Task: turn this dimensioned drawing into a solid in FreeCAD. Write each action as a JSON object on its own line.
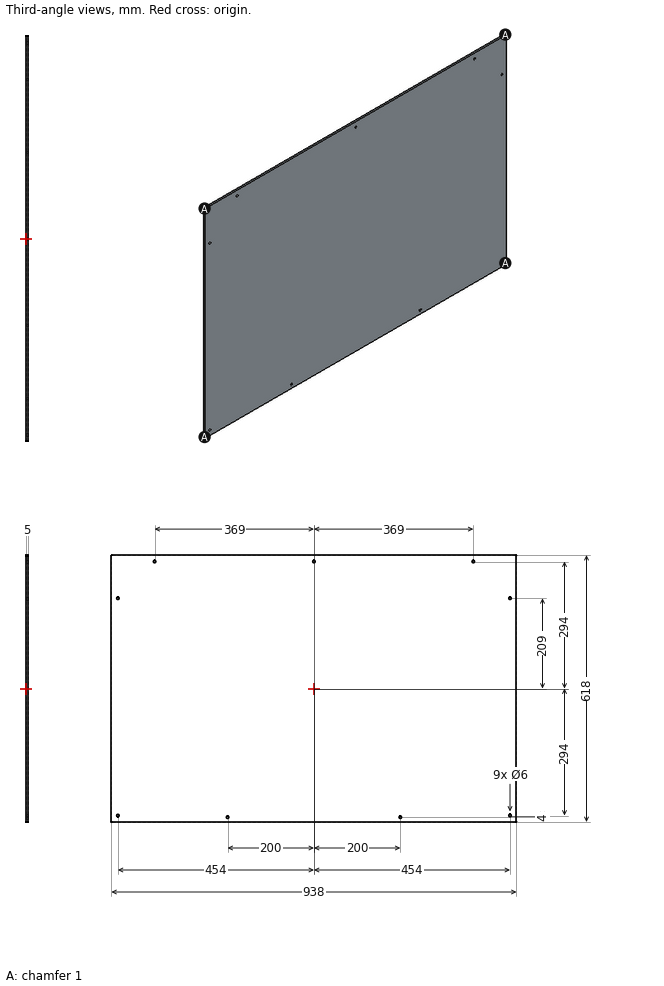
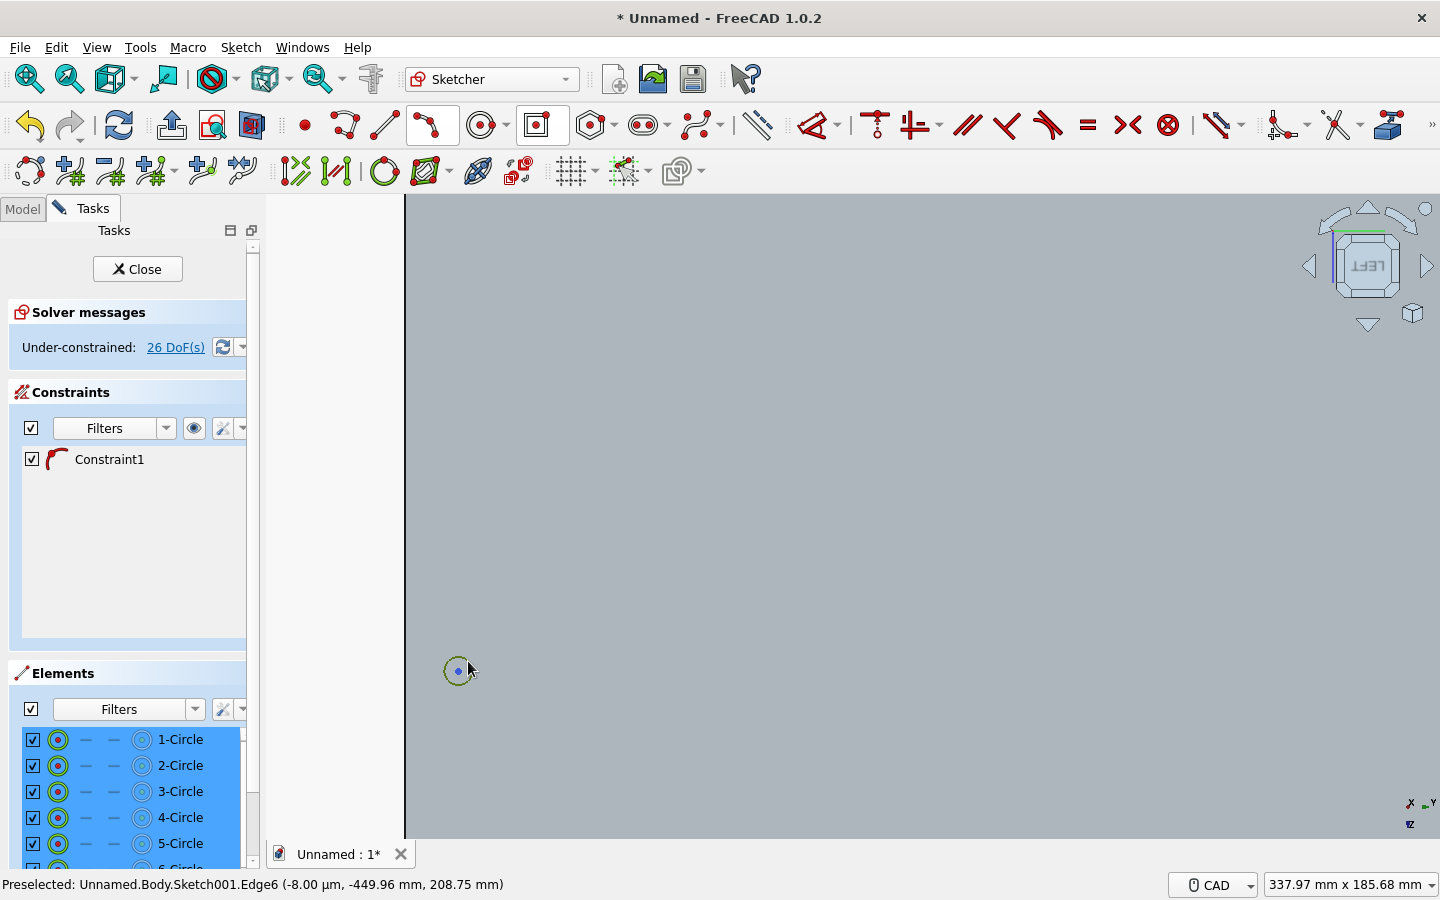
{"action": "scroll", "coordinate": [468, 664], "scroll_direction": "down", "scroll_amount": 8}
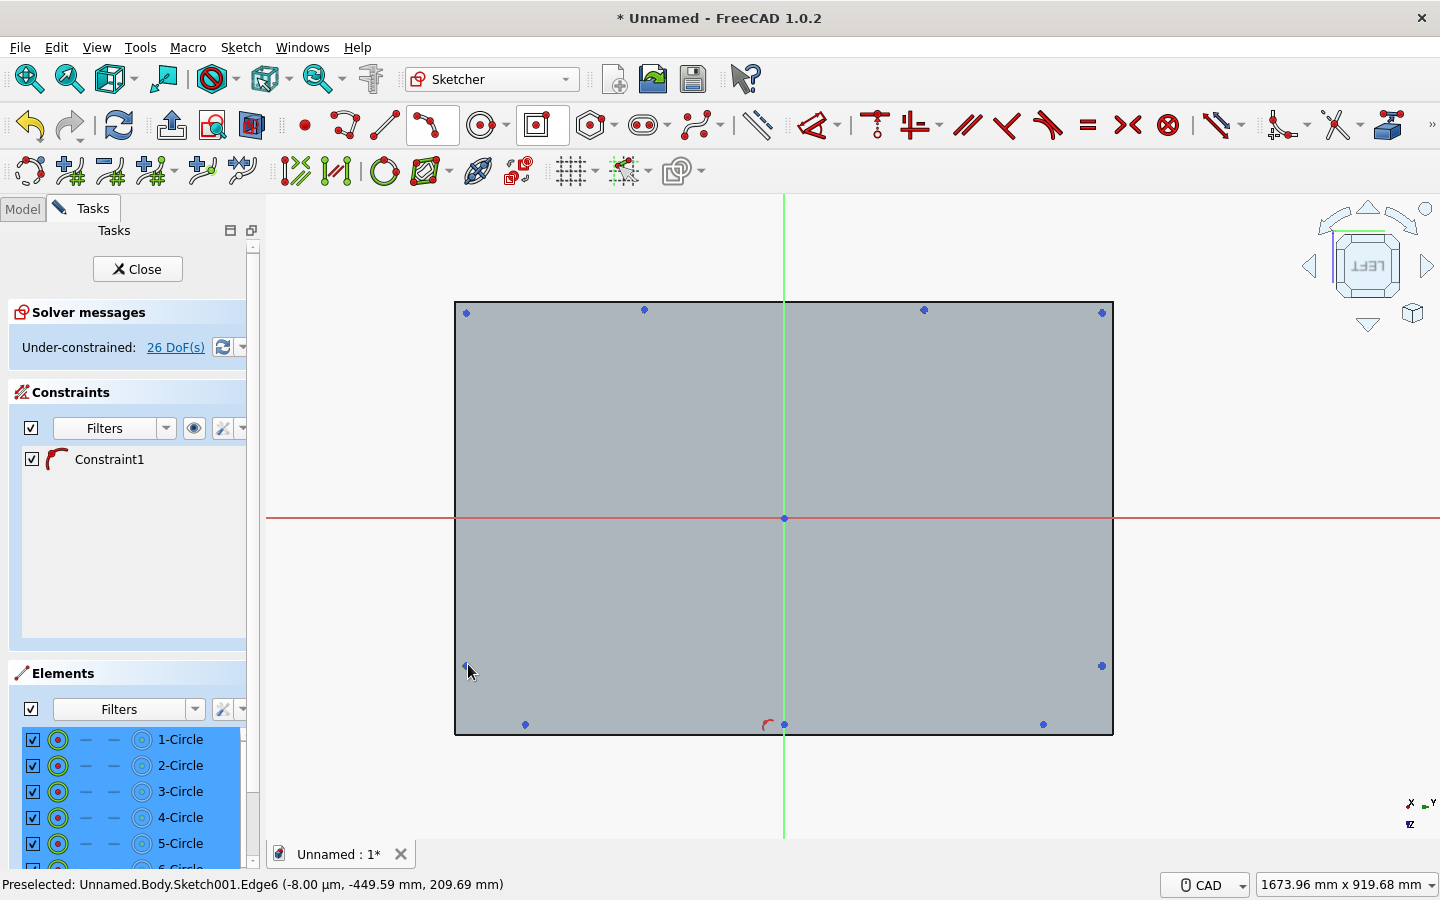
{"action": "scroll", "coordinate": [784, 723], "scroll_direction": "up", "scroll_amount": 9}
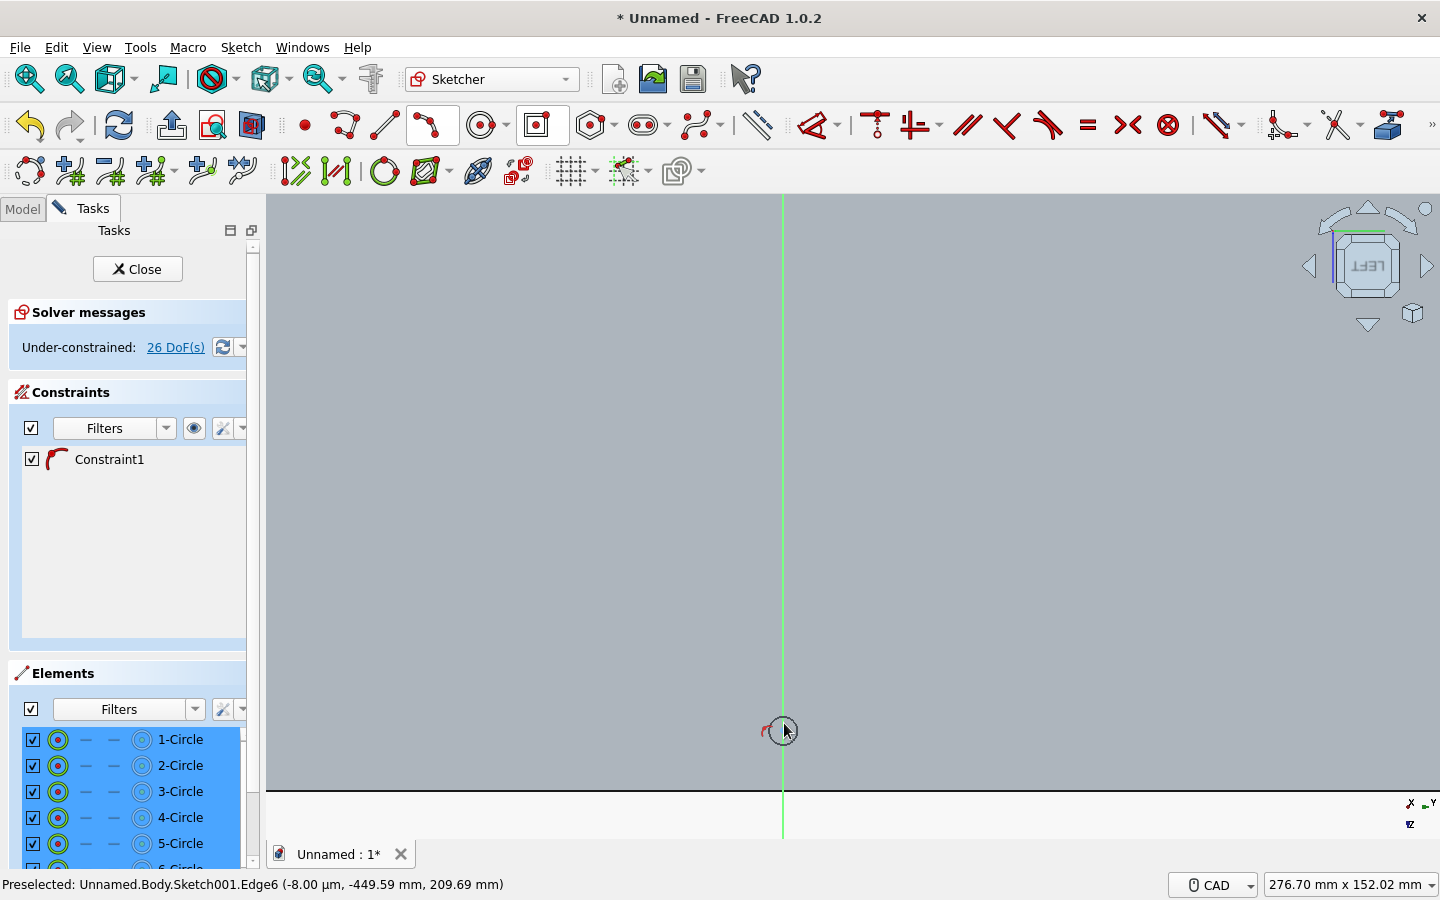
{"action": "left_click", "coordinate": [784, 717]}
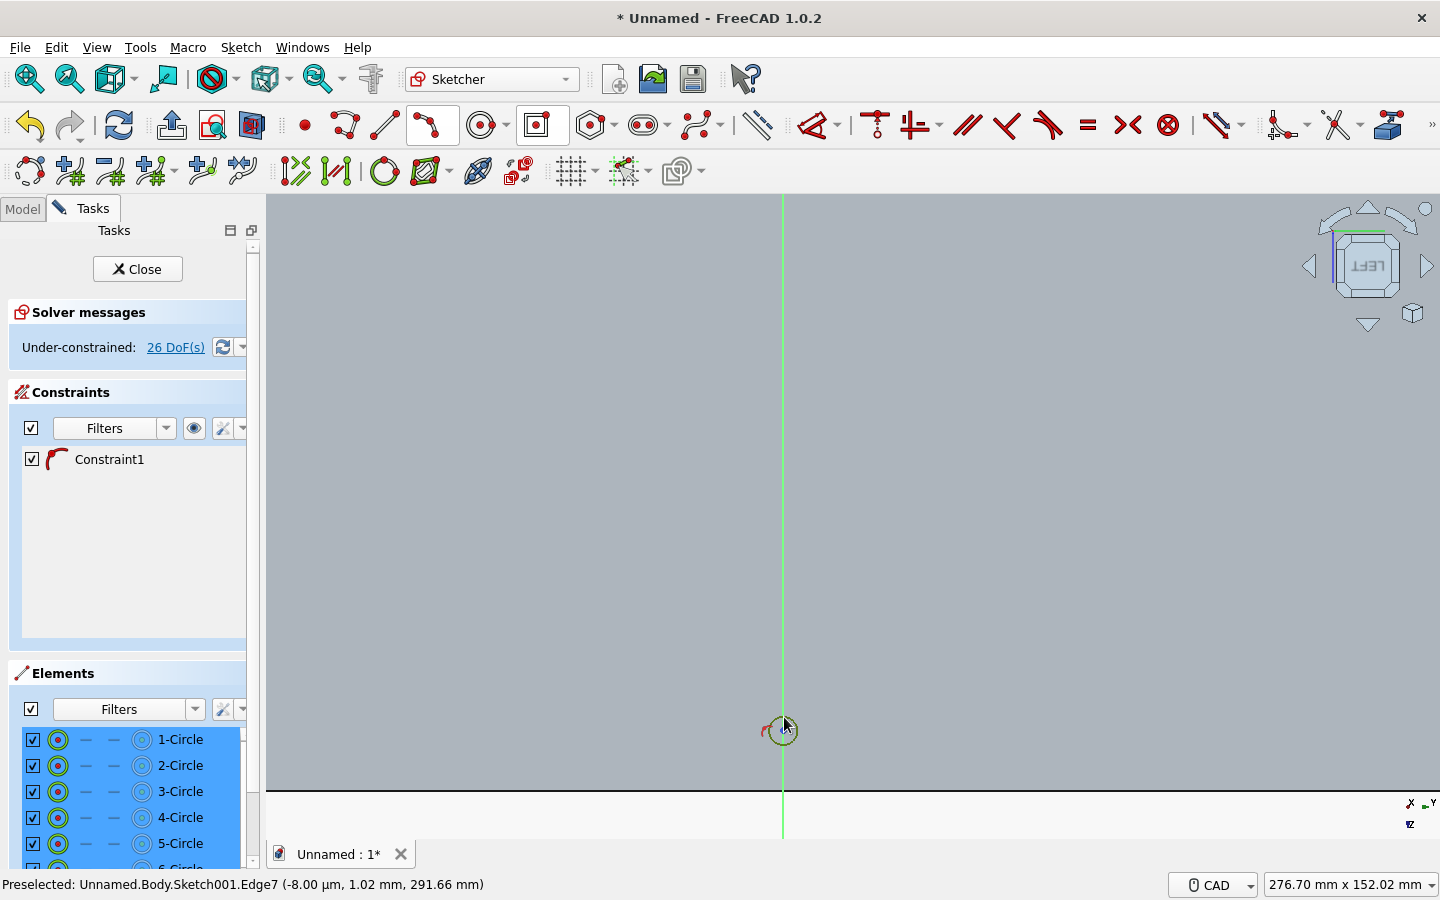
{"action": "scroll", "coordinate": [785, 723], "scroll_direction": "down", "scroll_amount": 9}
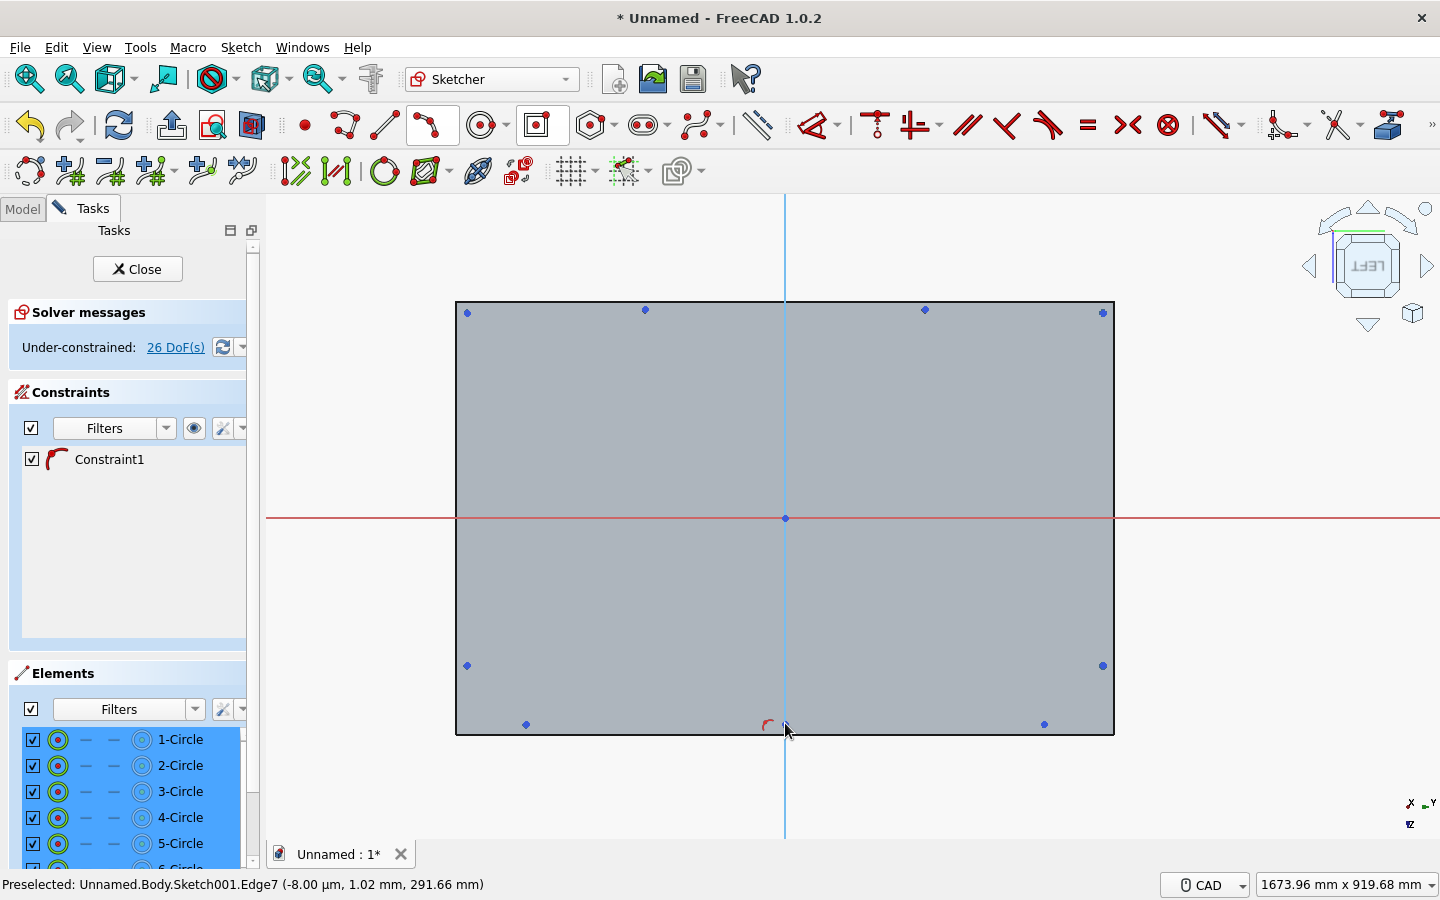
{"action": "scroll", "coordinate": [927, 308], "scroll_direction": "up", "scroll_amount": 8}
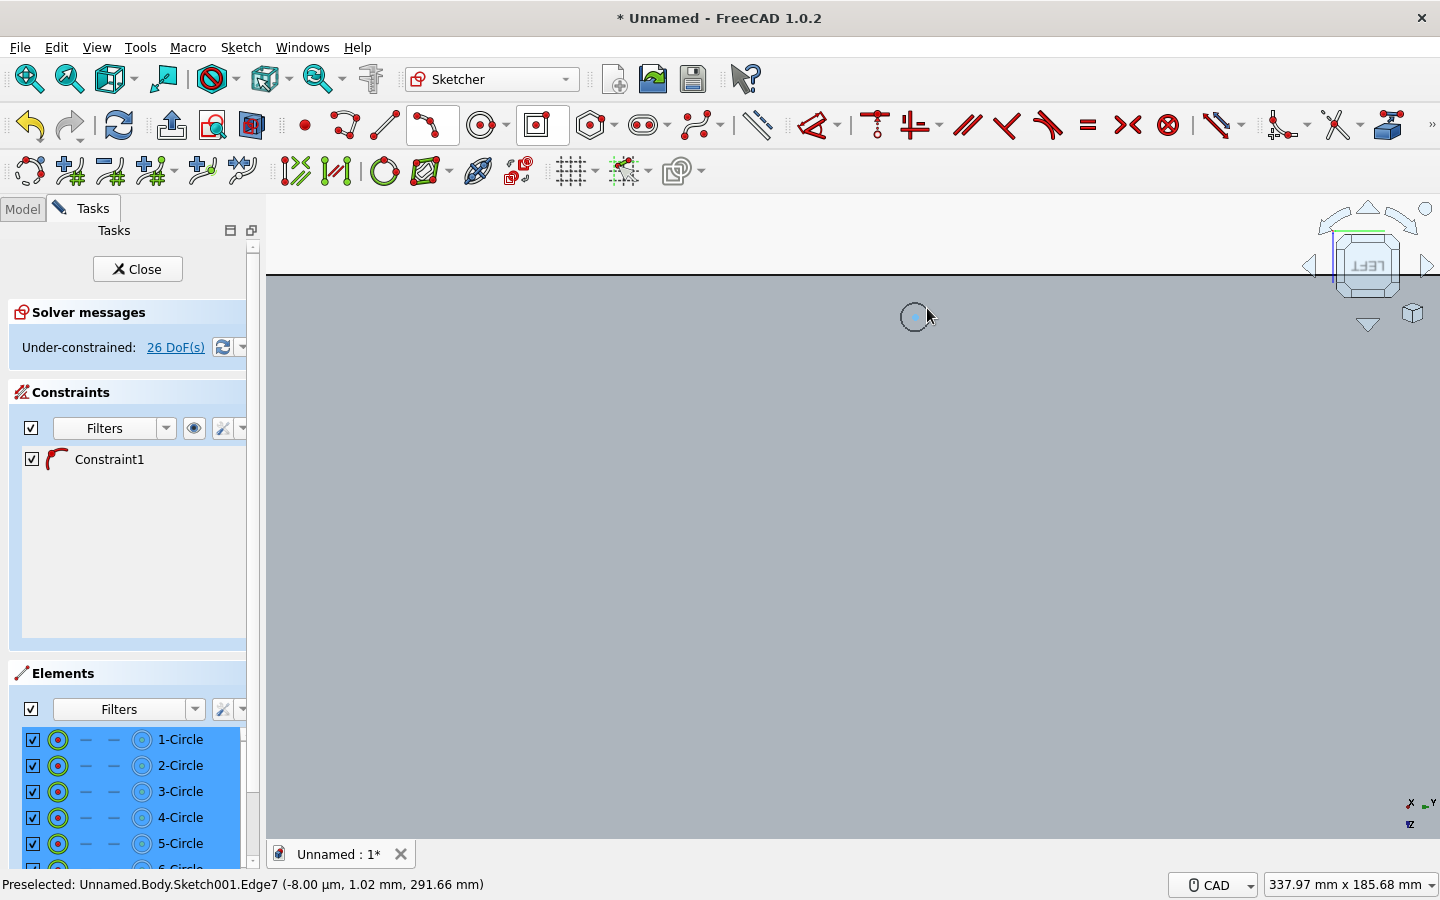
{"action": "left_click", "coordinate": [925, 307]}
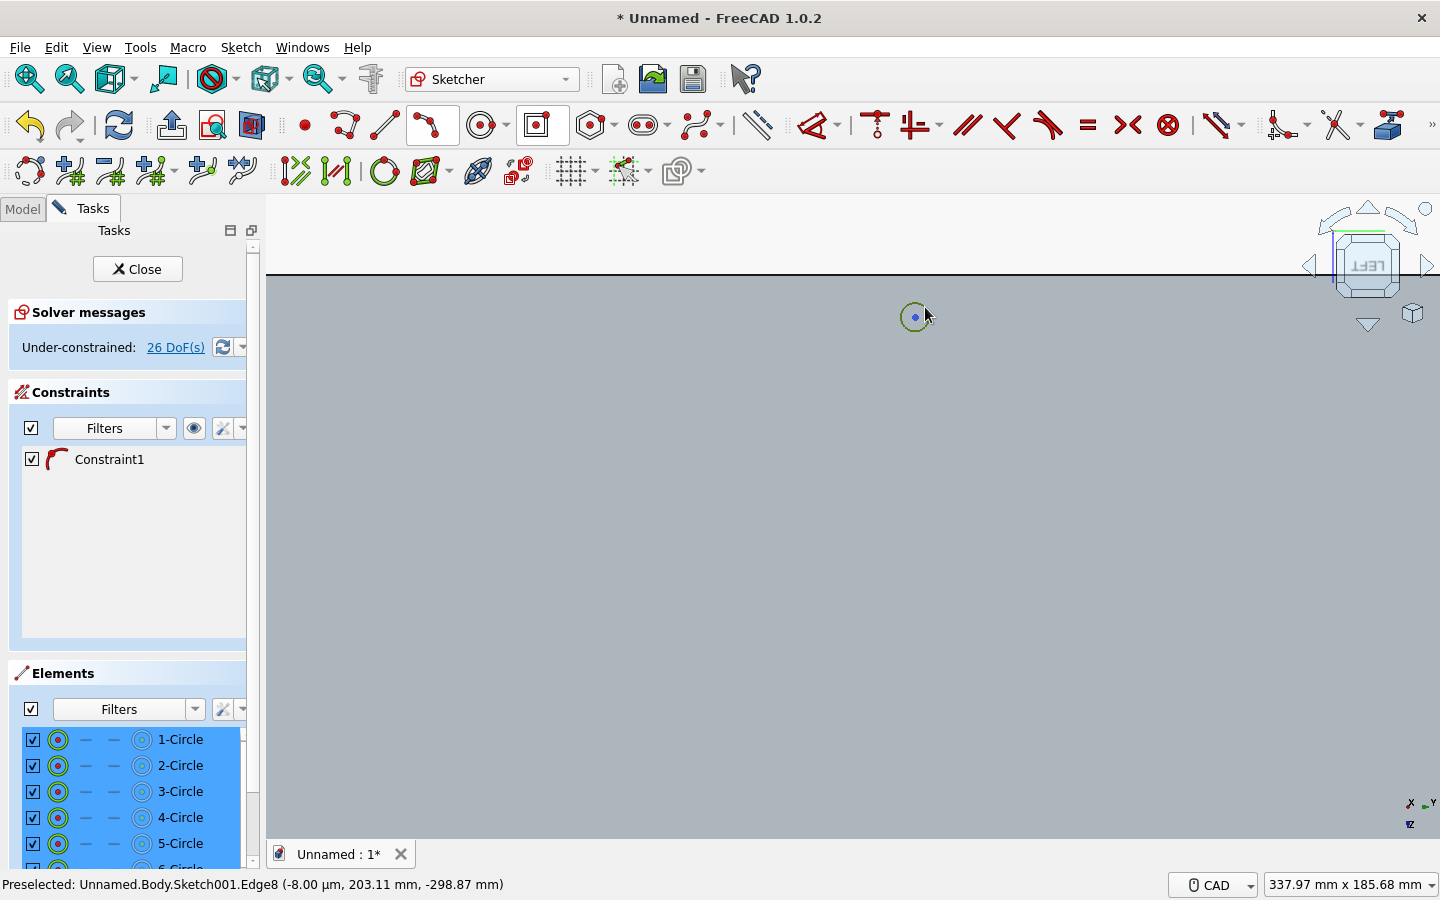
{"action": "scroll", "coordinate": [927, 308], "scroll_direction": "down", "scroll_amount": 8}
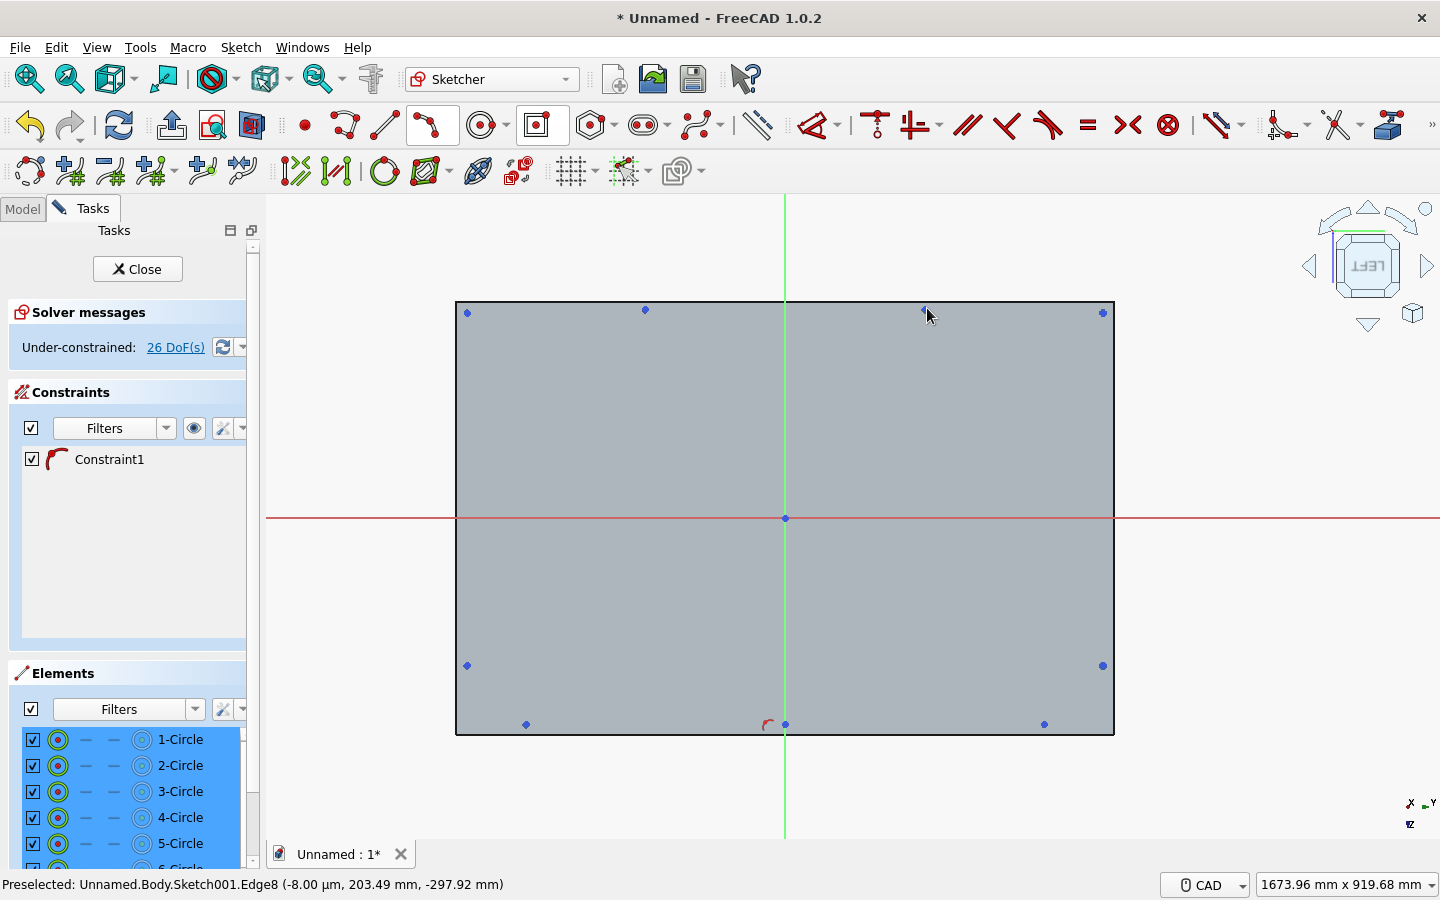
{"action": "scroll", "coordinate": [647, 308], "scroll_direction": "up", "scroll_amount": 9}